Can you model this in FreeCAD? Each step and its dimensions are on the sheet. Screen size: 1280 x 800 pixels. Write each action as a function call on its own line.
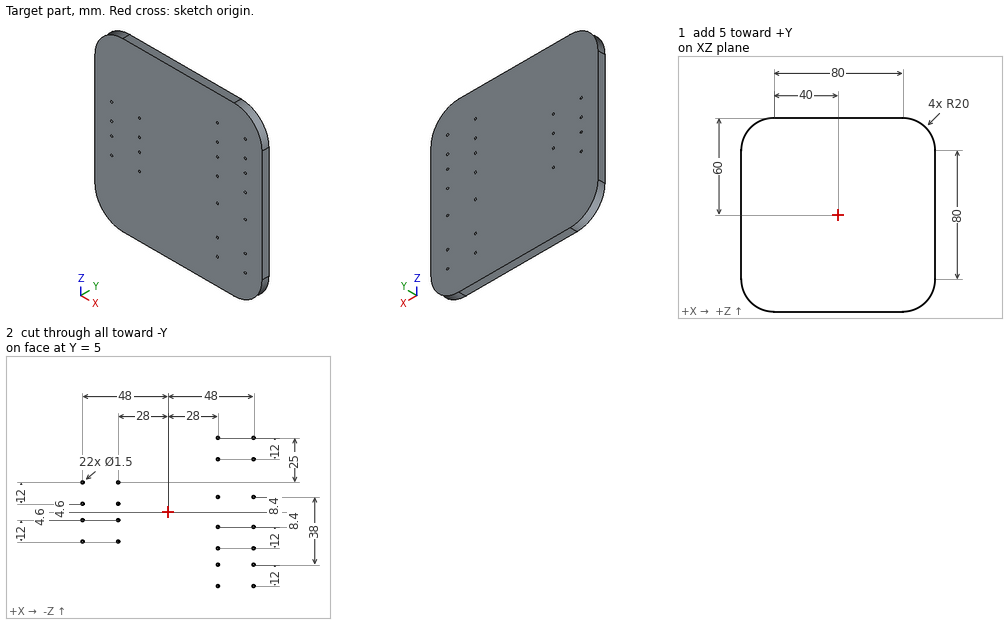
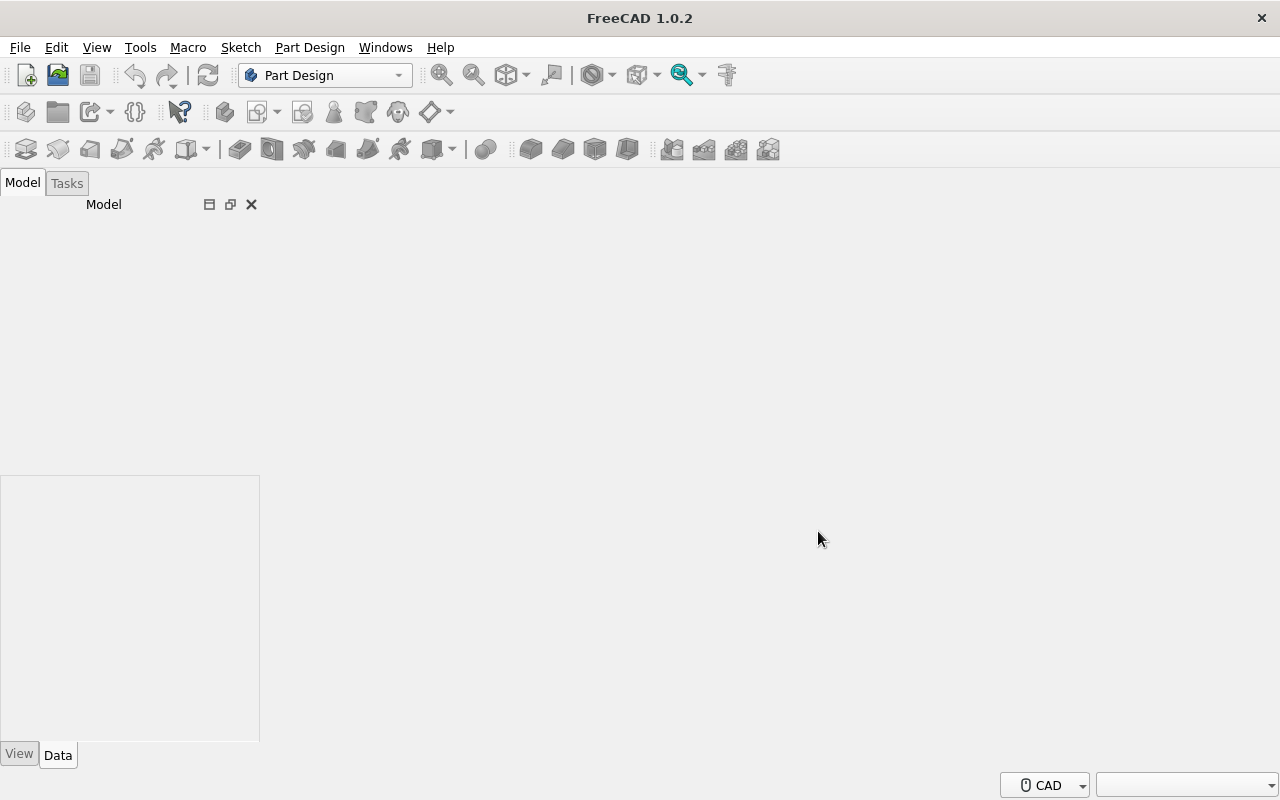
click(26, 76)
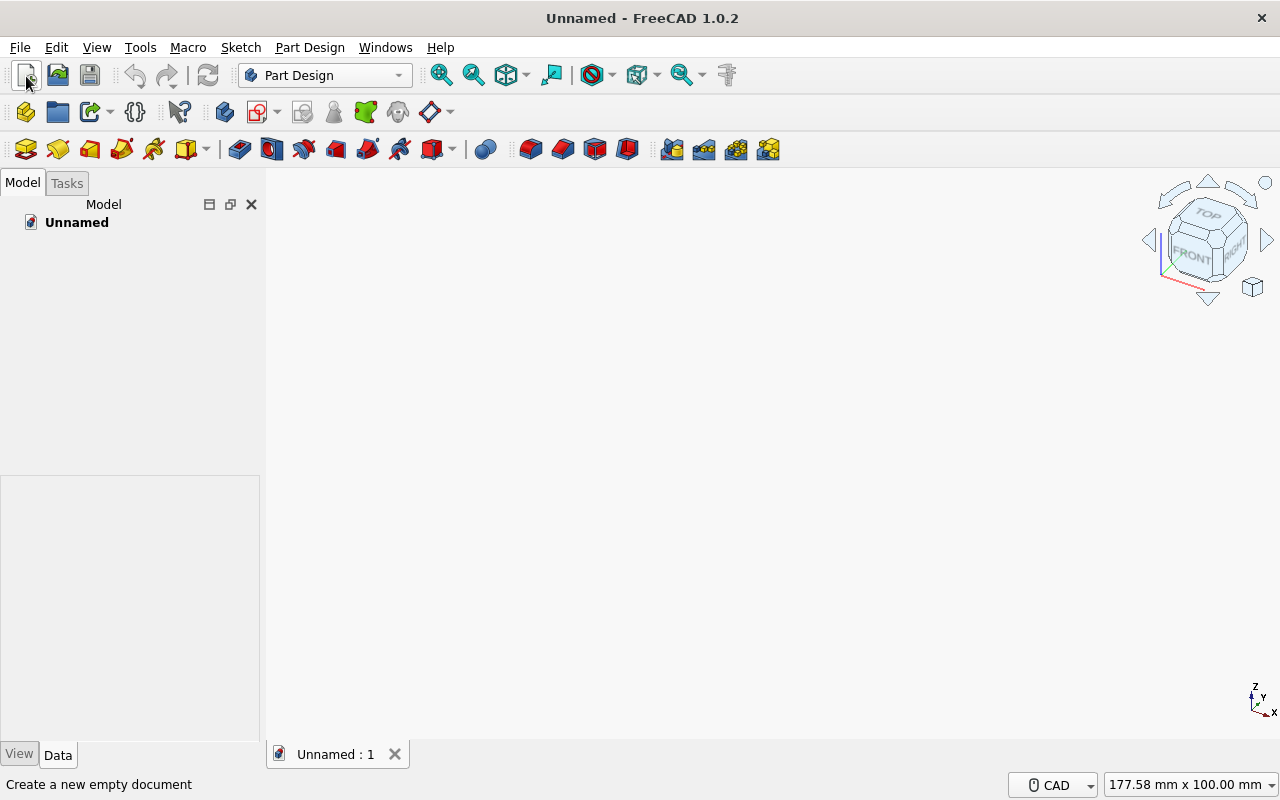
click(258, 112)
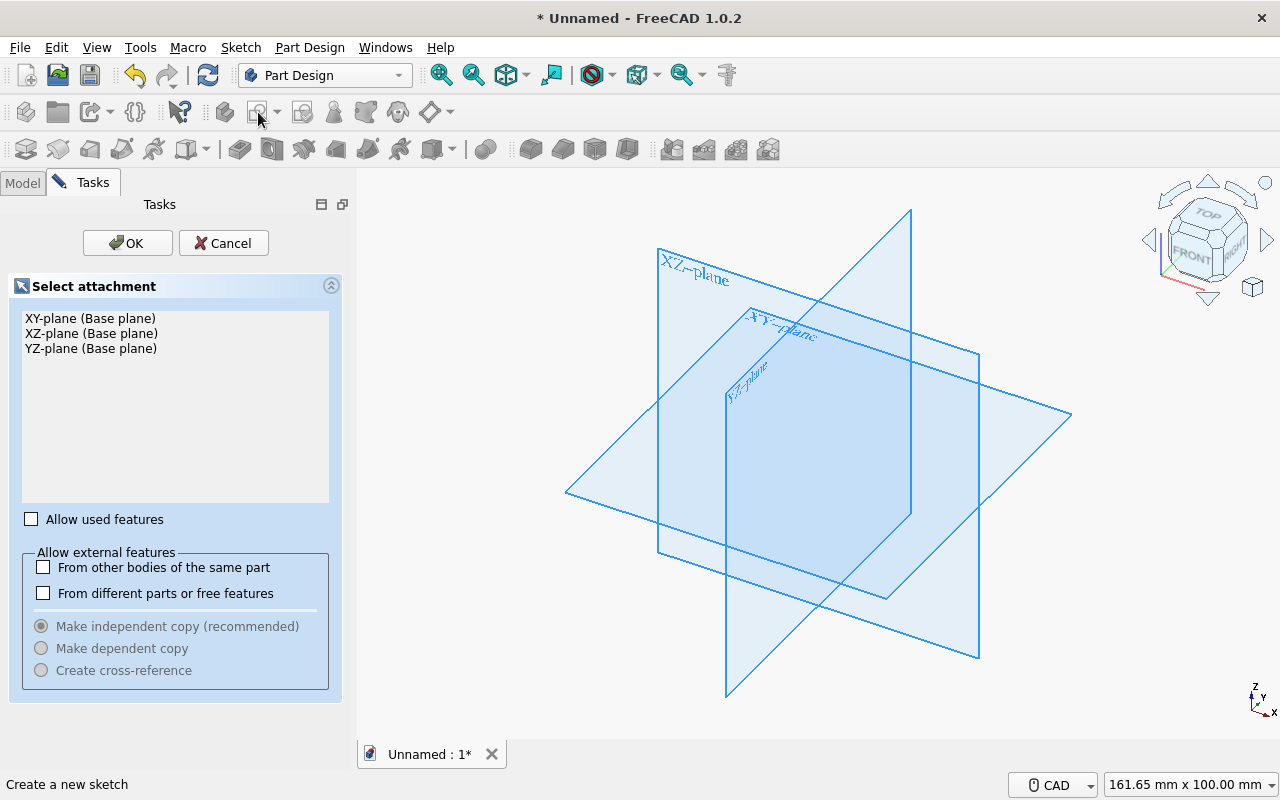
click(82, 334)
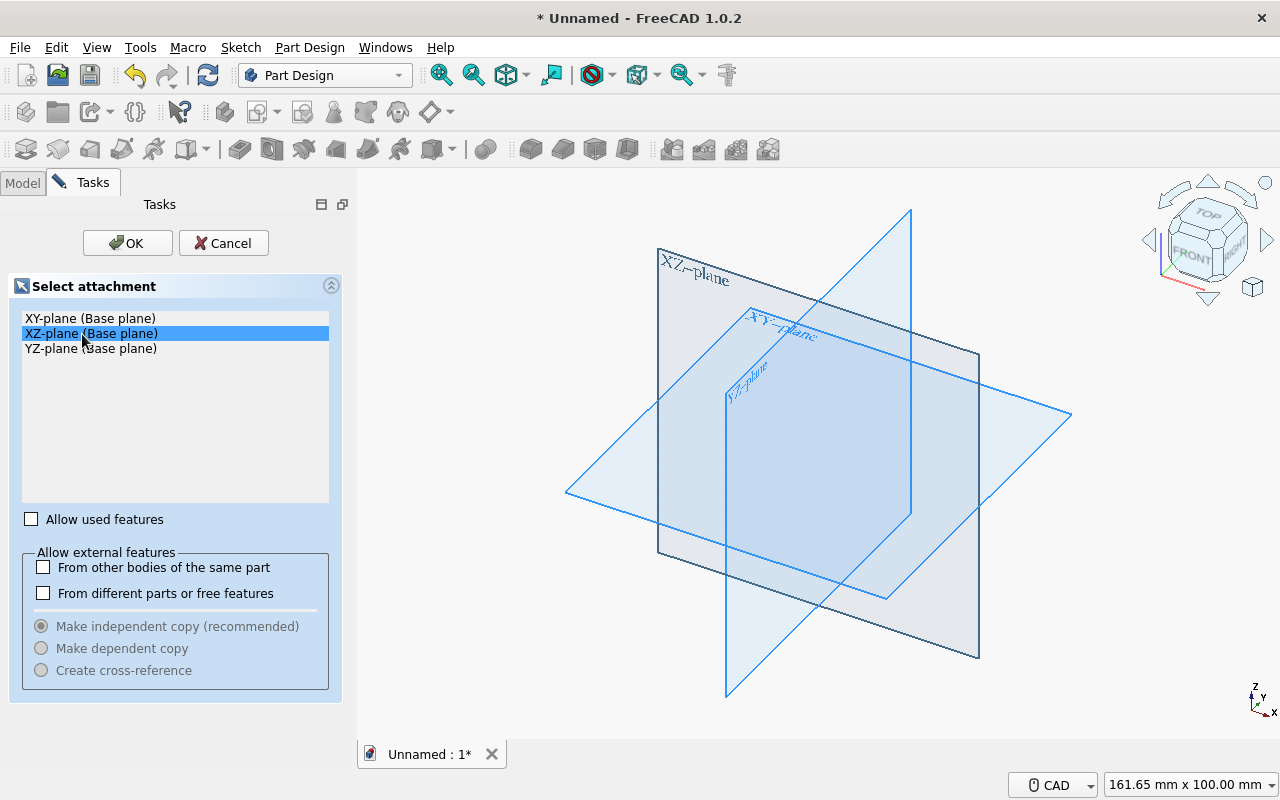
click(128, 243)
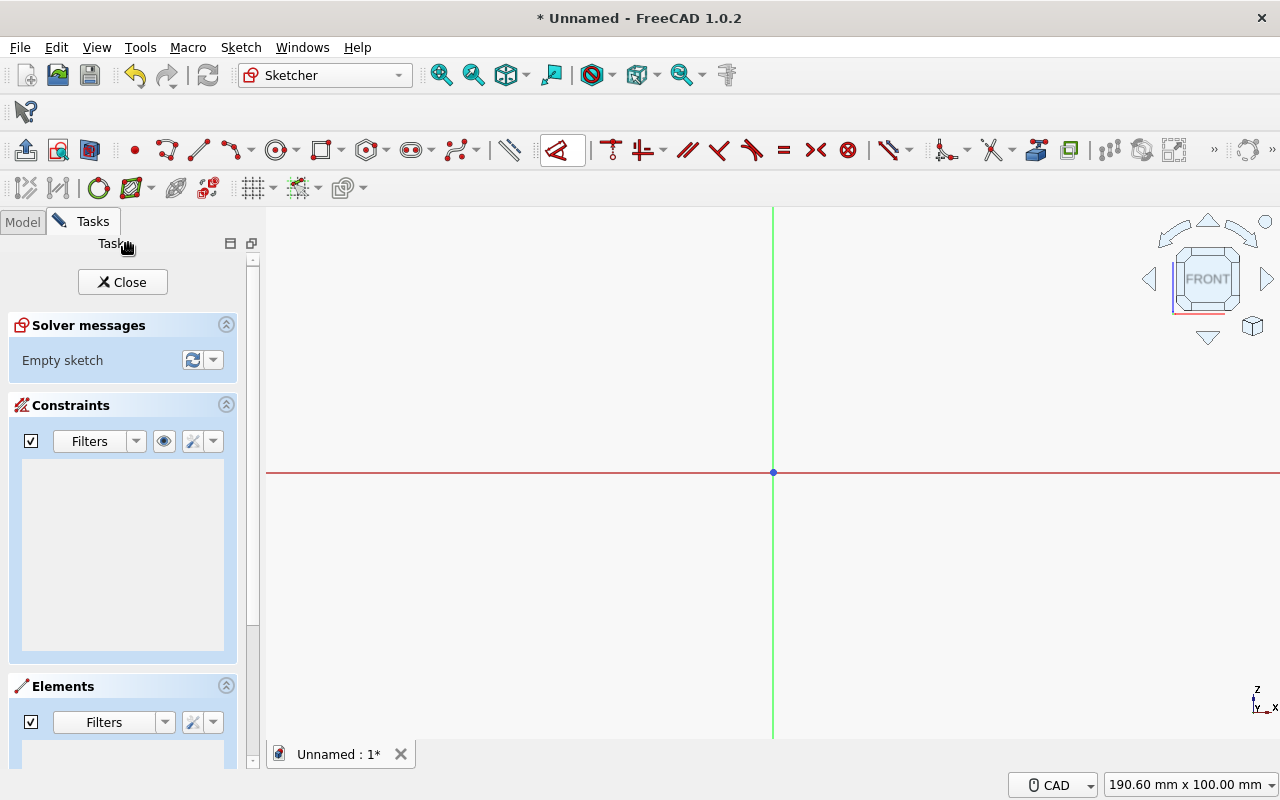
scroll(621, 473, down, 3)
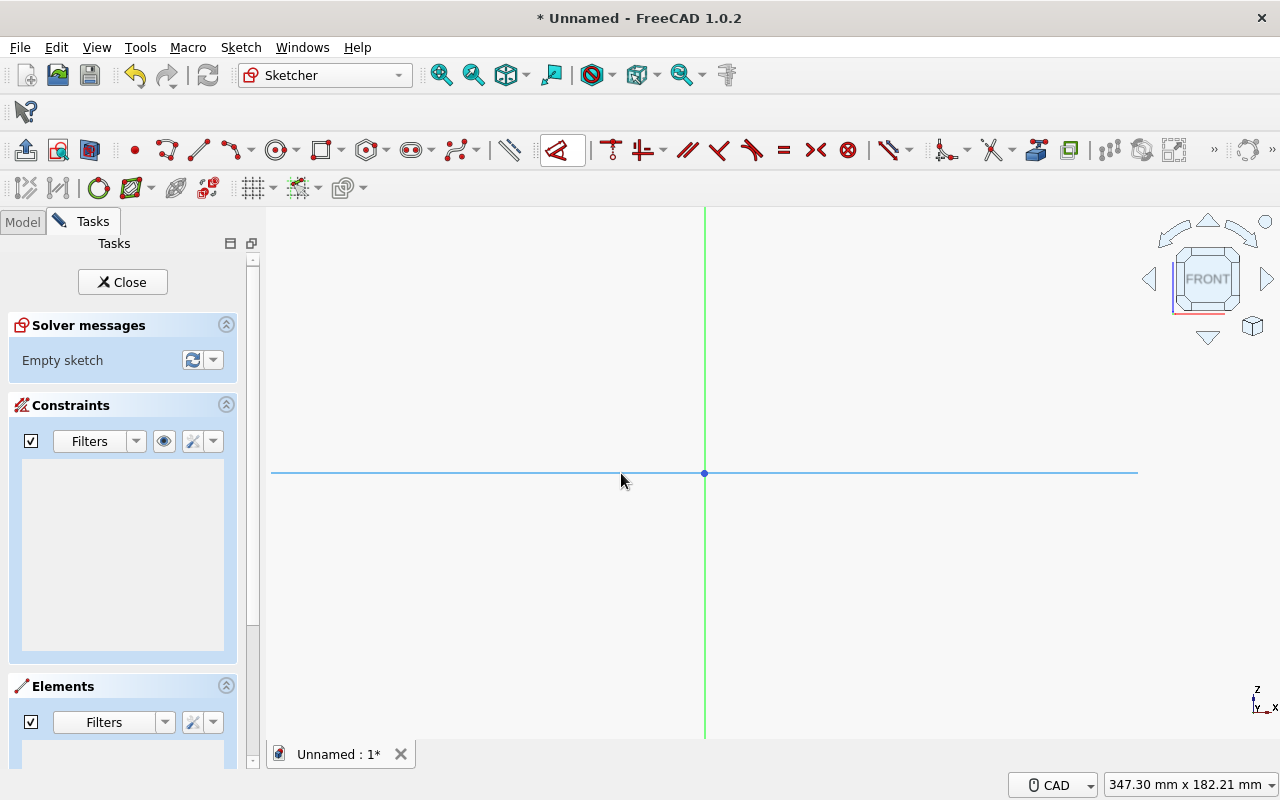
click(200, 150)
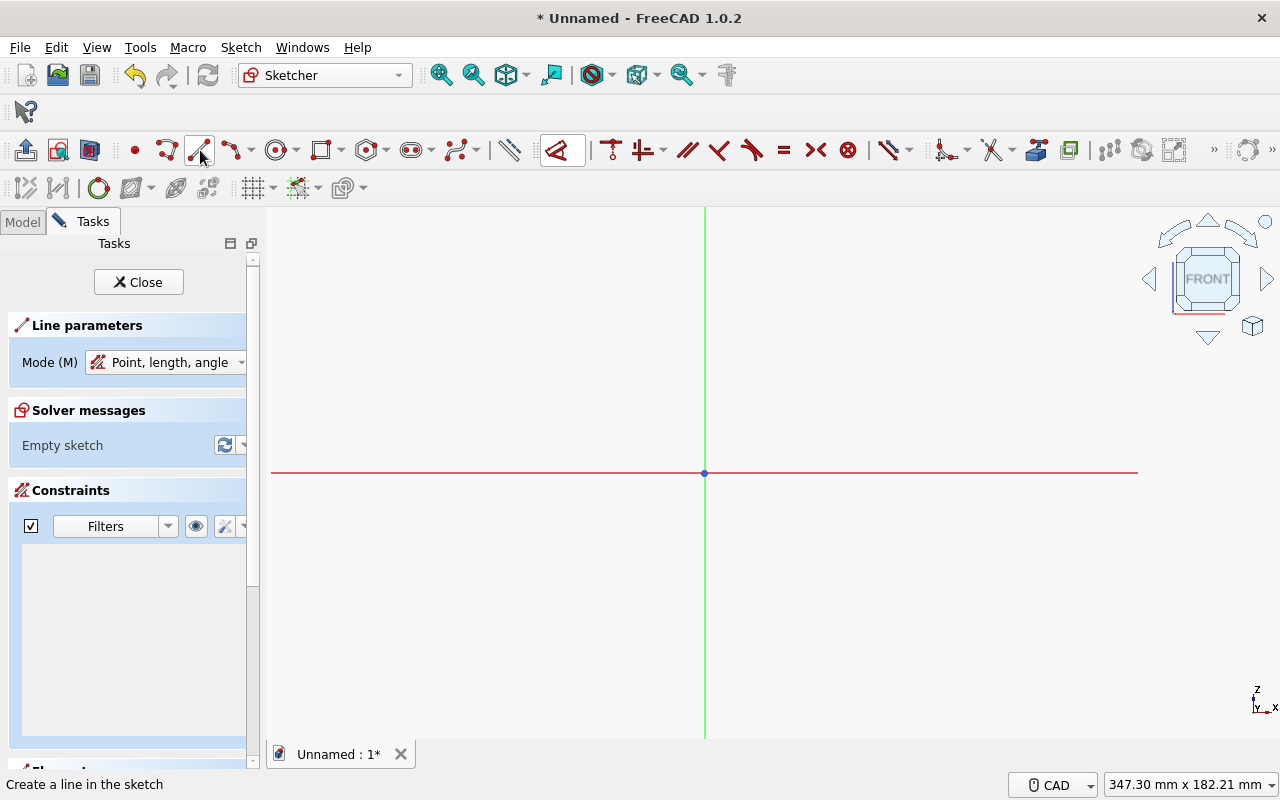
click(588, 298)
click(821, 298)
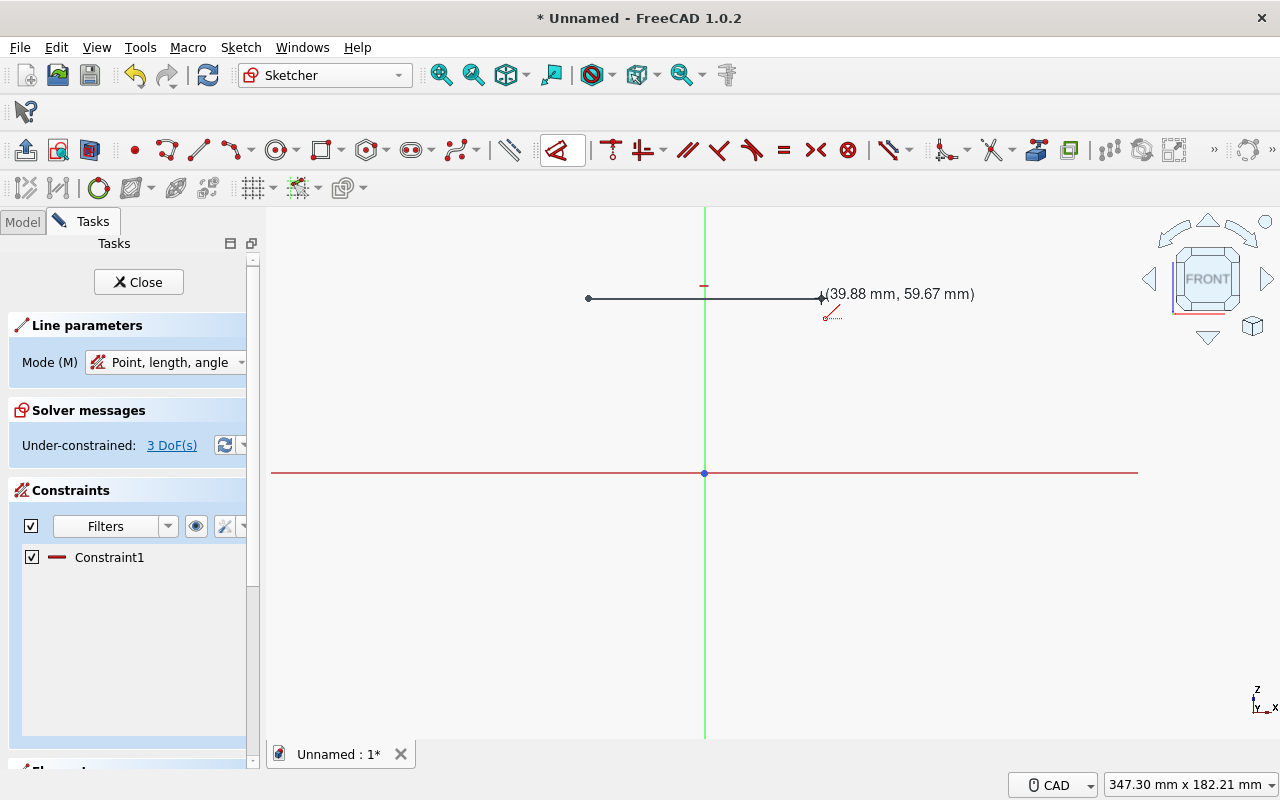
click(880, 356)
click(880, 590)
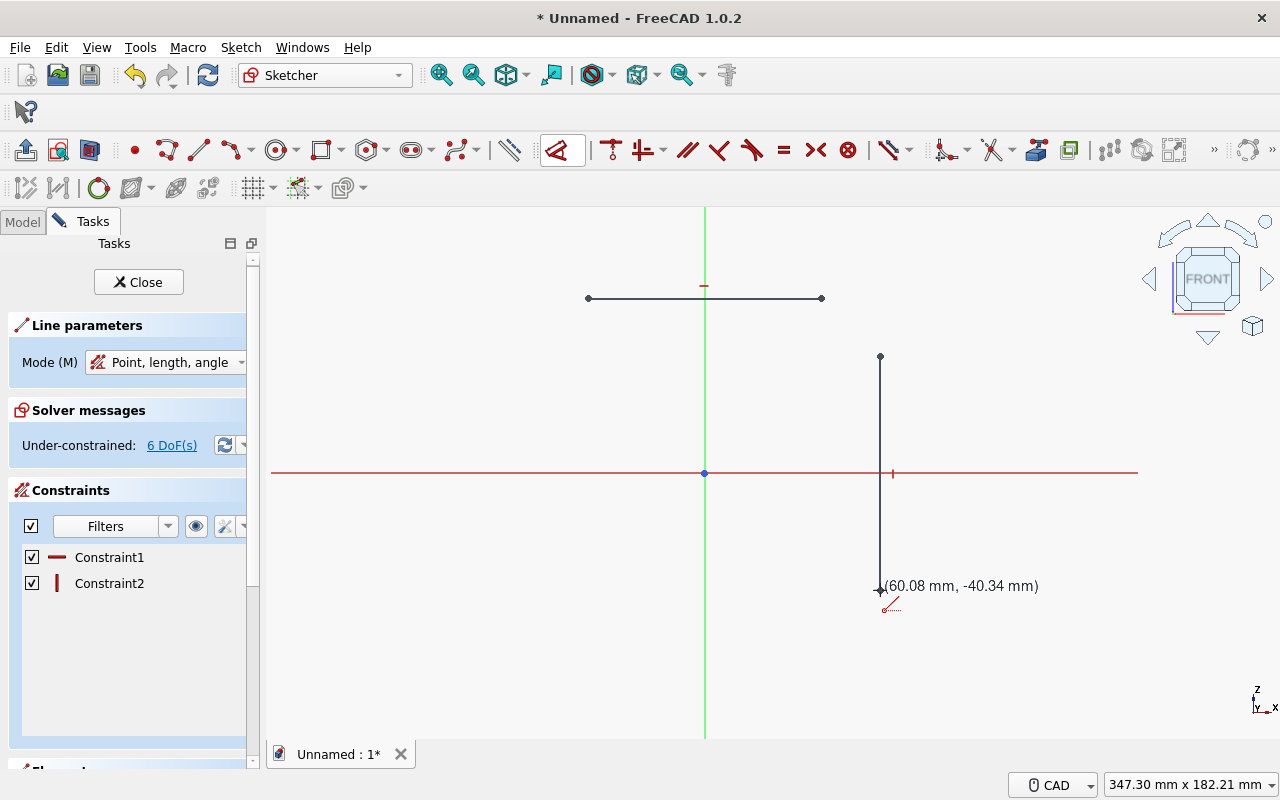
click(821, 648)
click(588, 648)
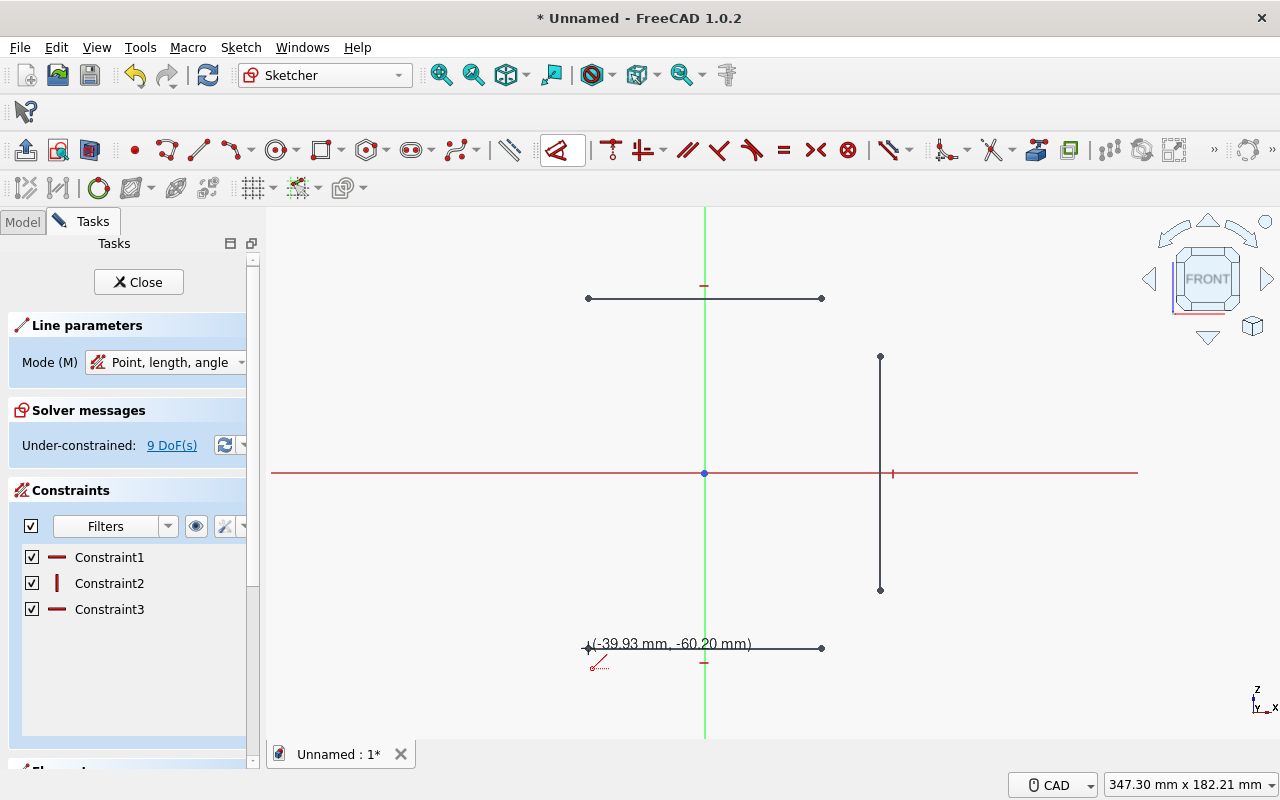
click(529, 590)
click(529, 356)